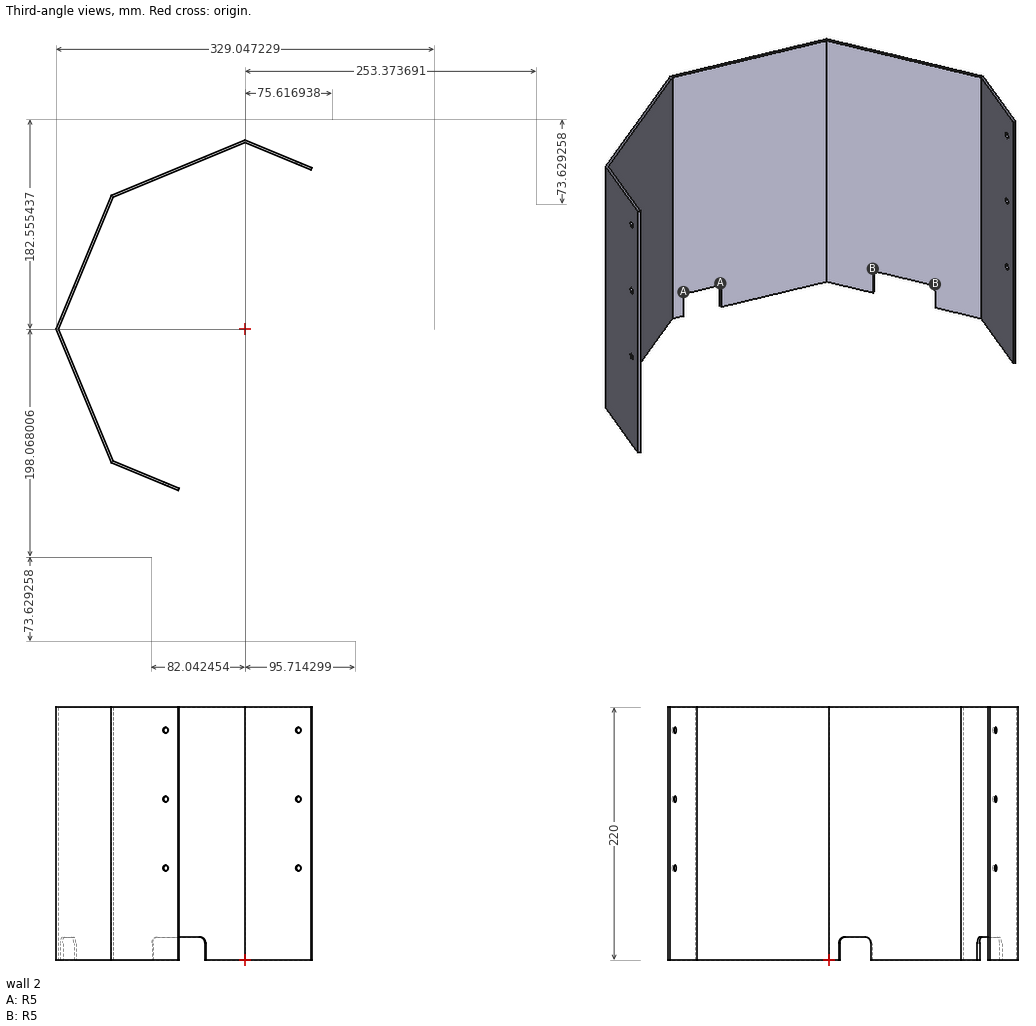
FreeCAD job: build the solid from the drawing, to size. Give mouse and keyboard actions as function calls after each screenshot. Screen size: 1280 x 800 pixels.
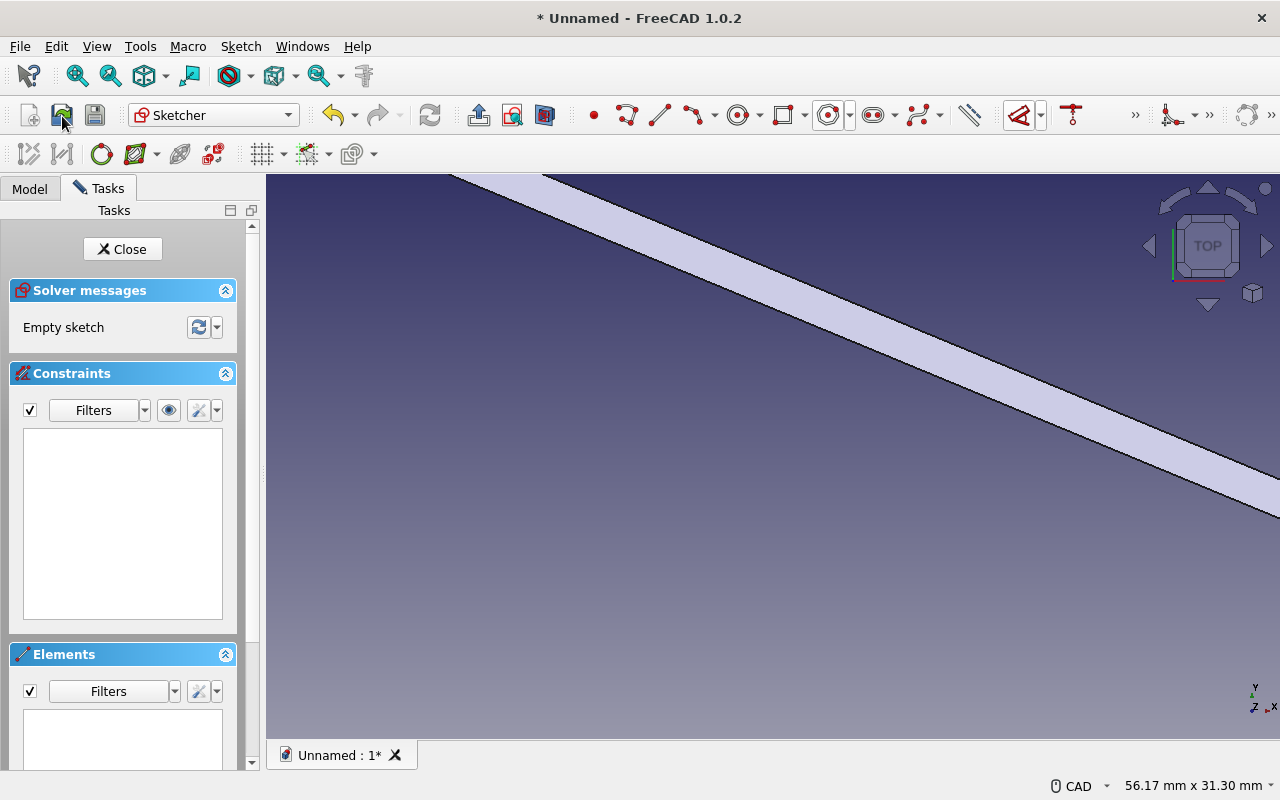
scroll(654, 283, down, 15)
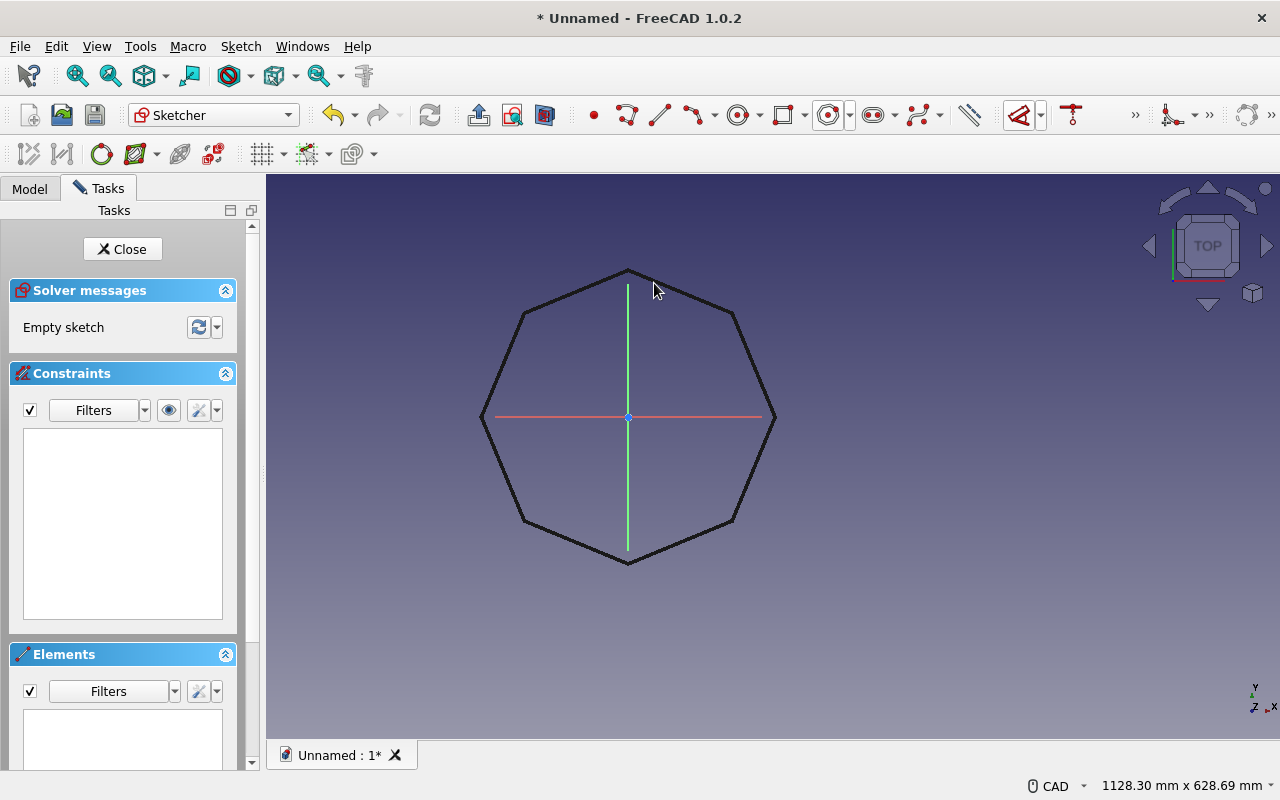
click(627, 116)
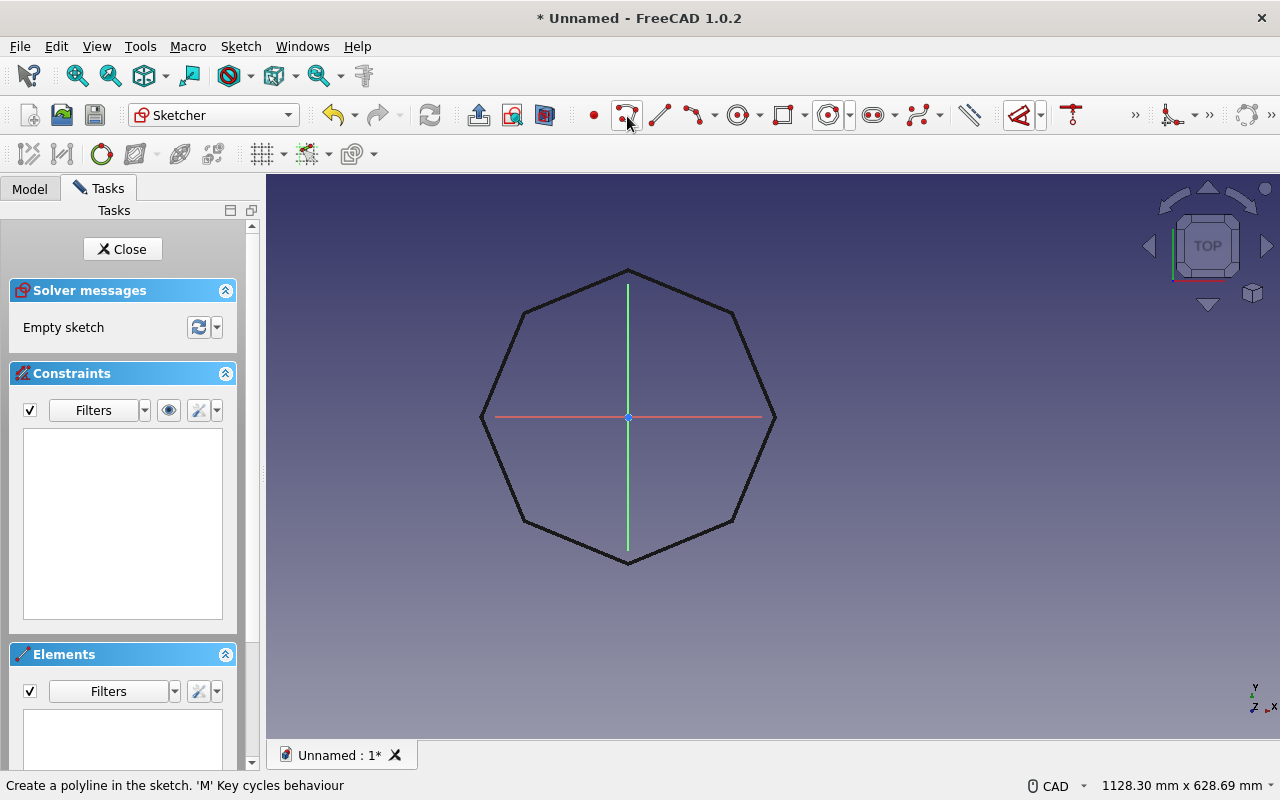
click(696, 253)
click(555, 595)
click(714, 661)
click(856, 319)
click(696, 254)
key(Escape)
key(Escape)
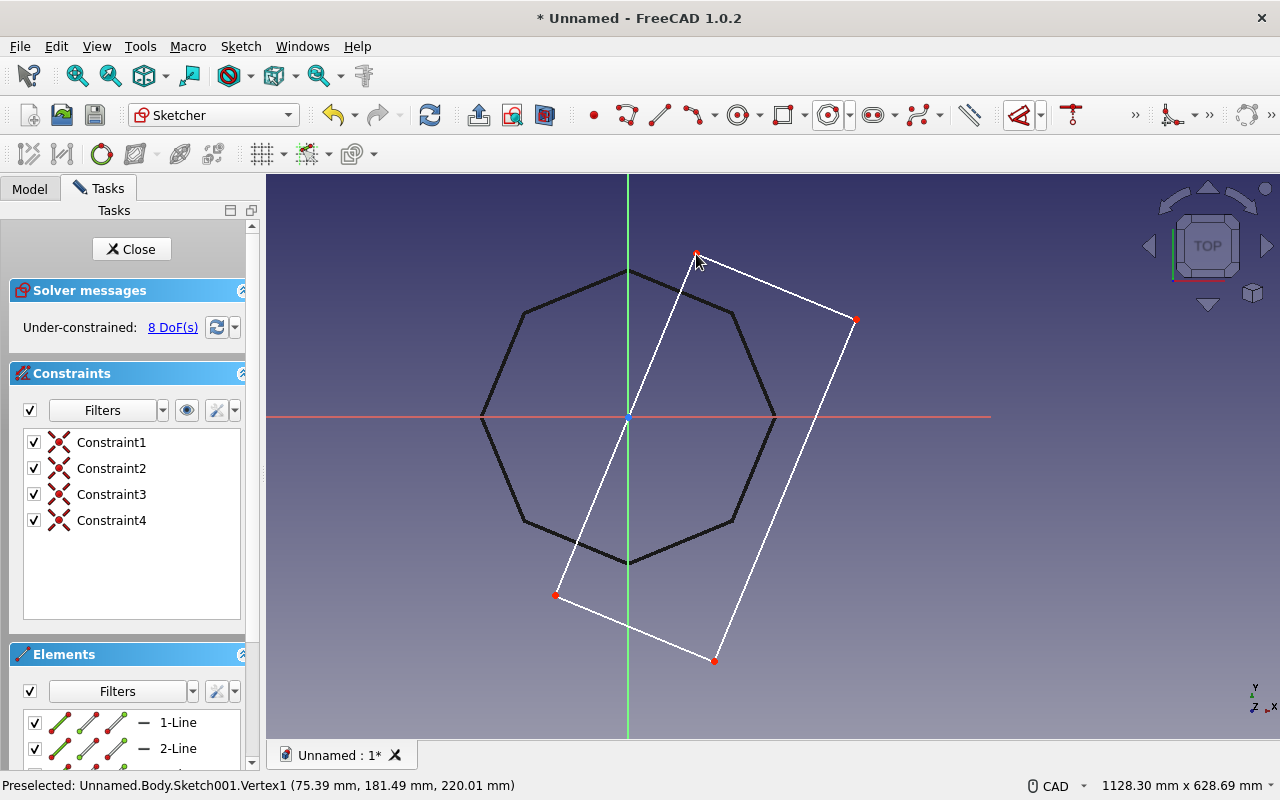
click(696, 254)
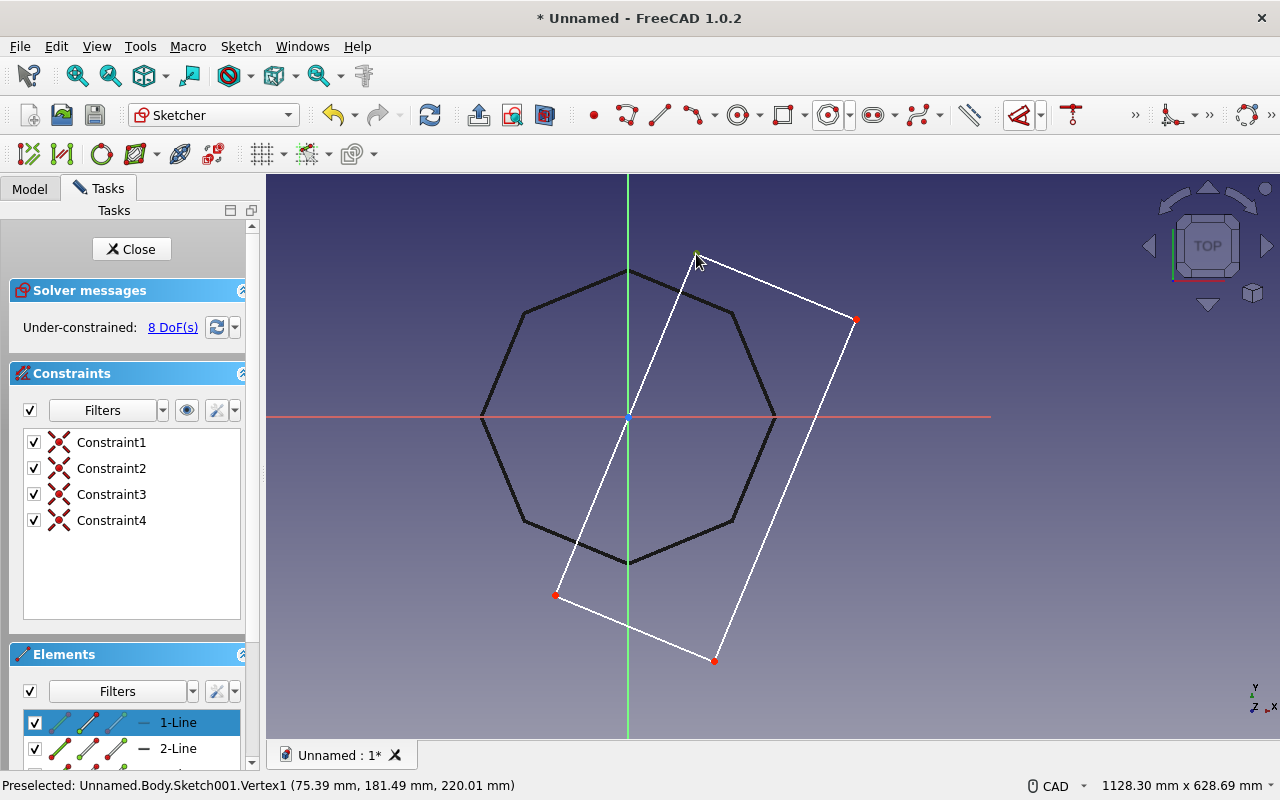
key(l)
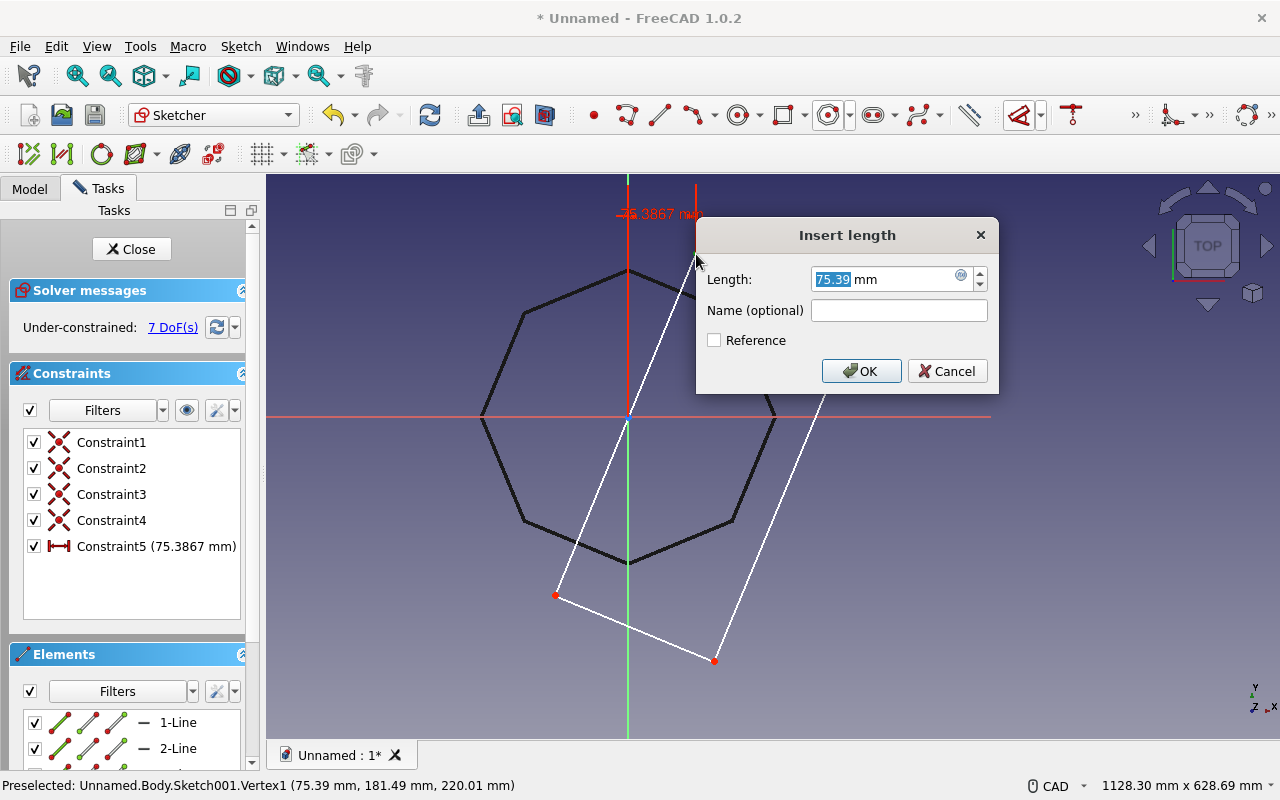
text(75.616938)
key(Return)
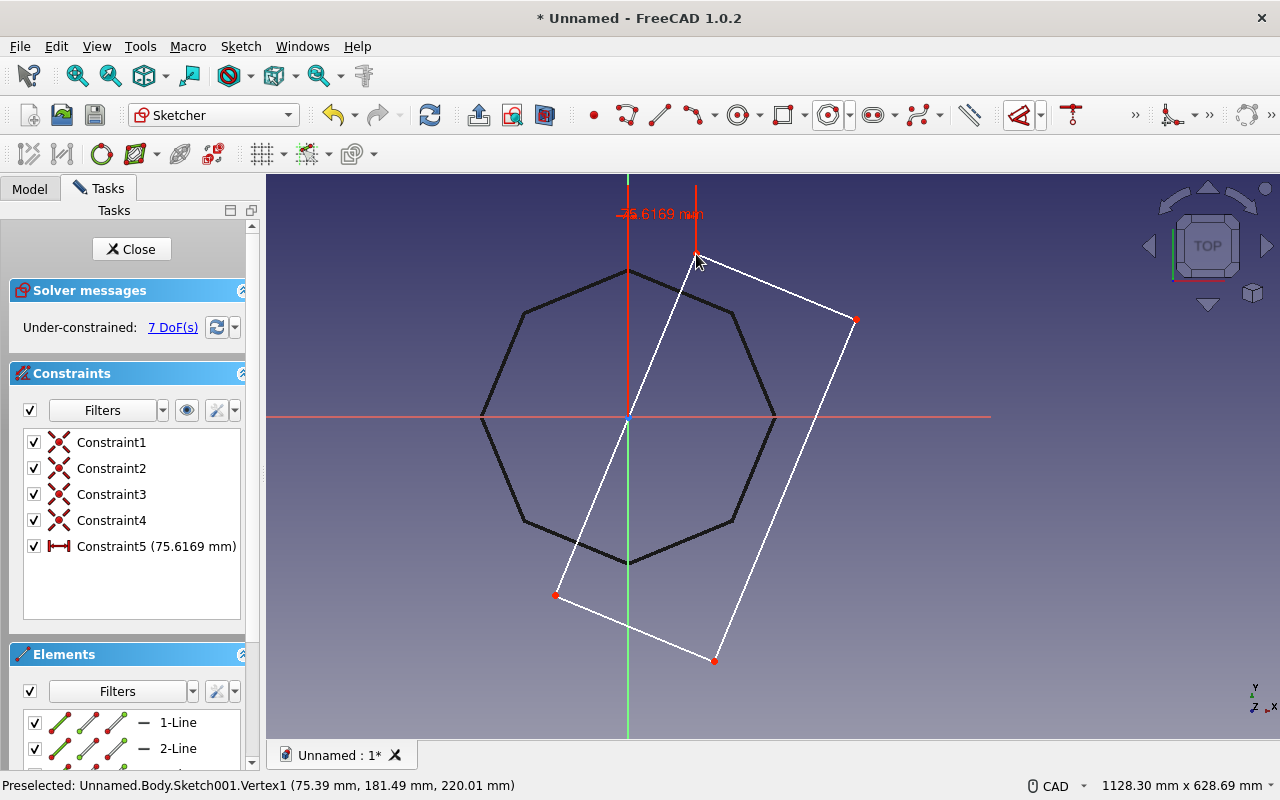
click(555, 596)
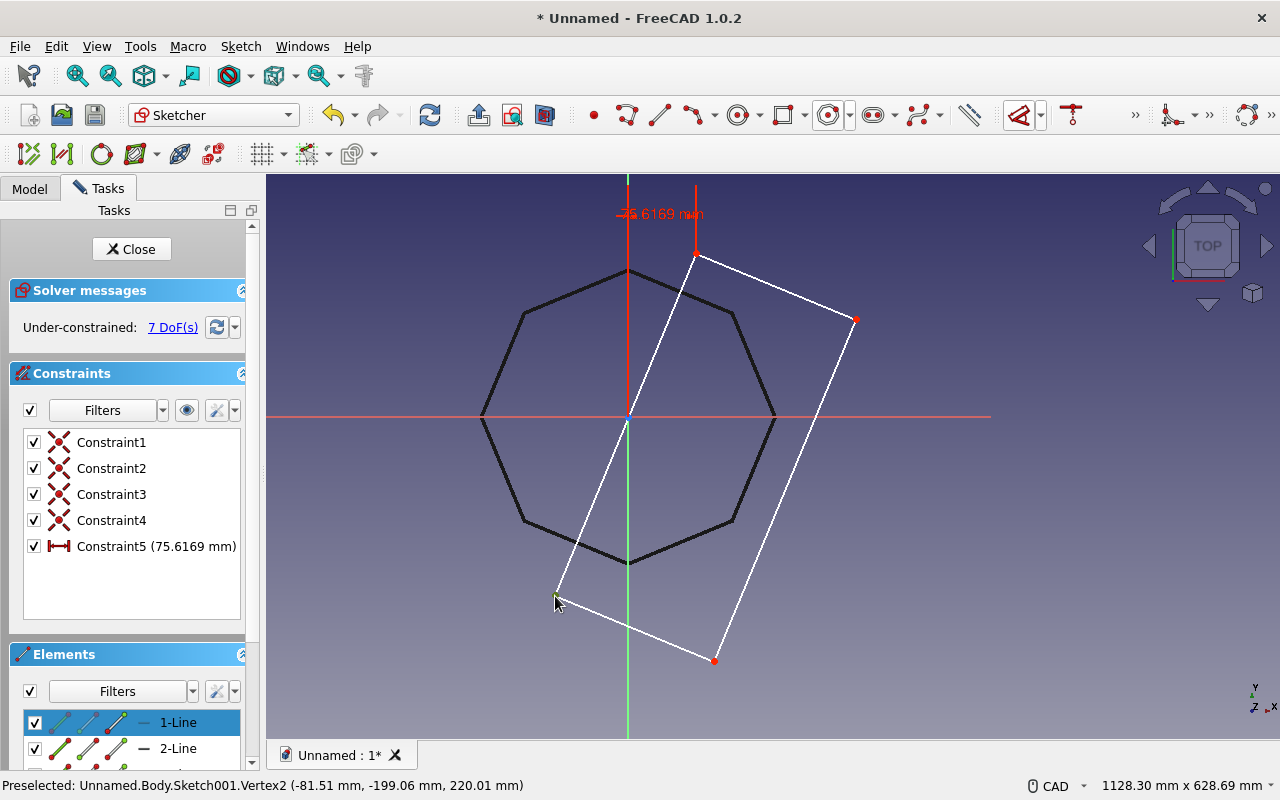
key(l)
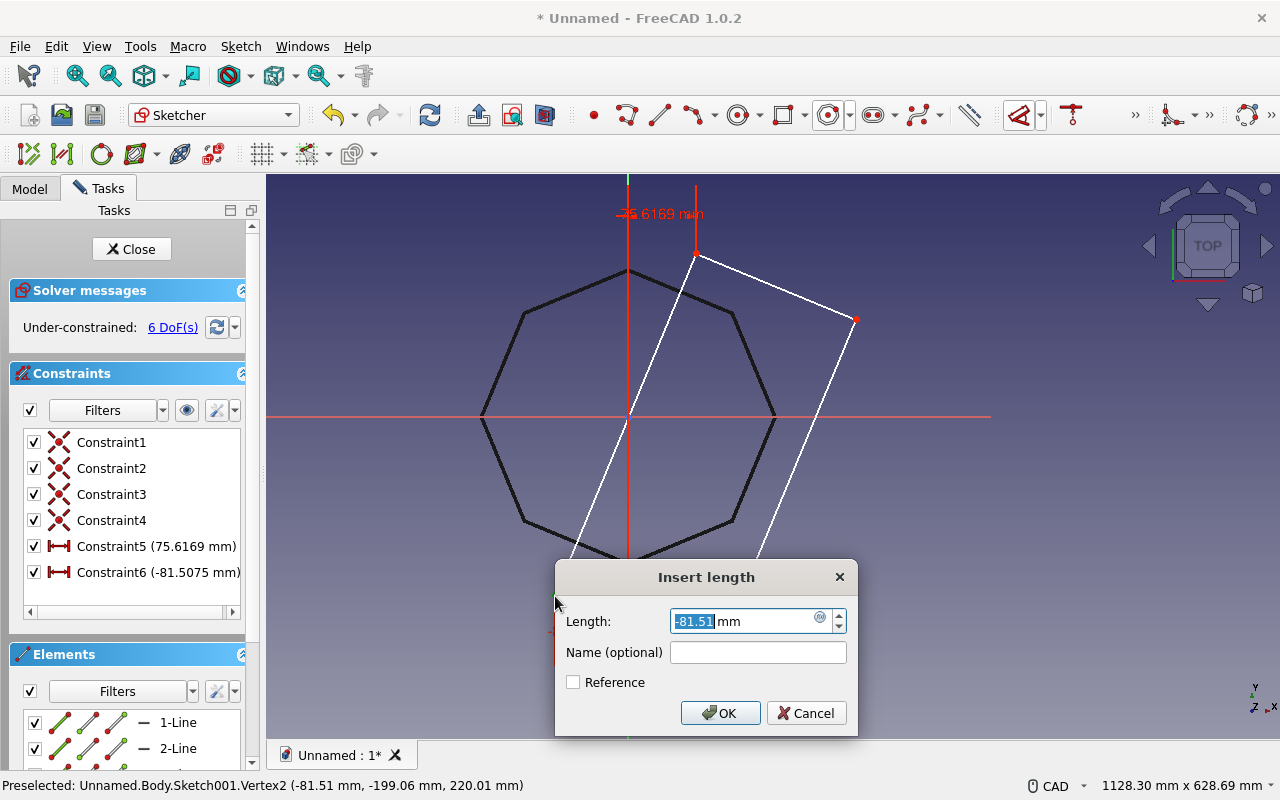
text(-82.042454)
key(Return)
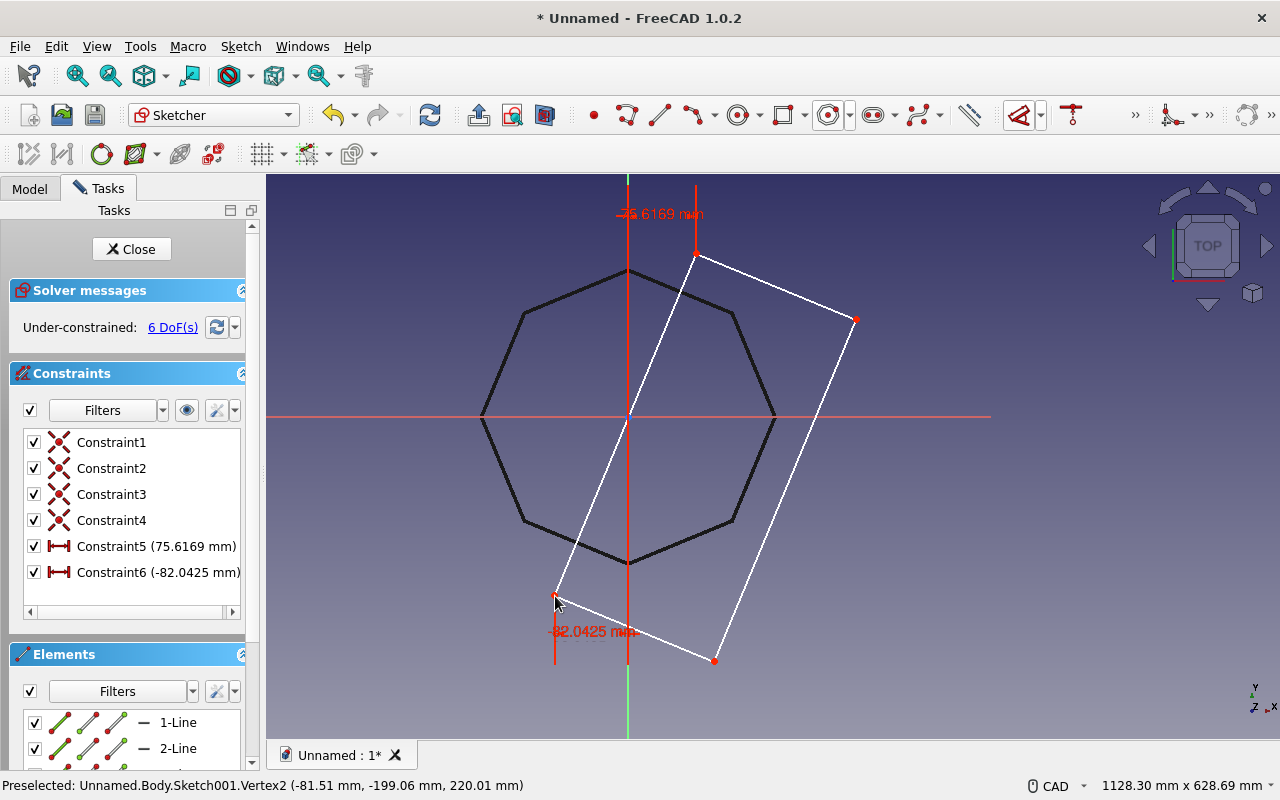
click(714, 662)